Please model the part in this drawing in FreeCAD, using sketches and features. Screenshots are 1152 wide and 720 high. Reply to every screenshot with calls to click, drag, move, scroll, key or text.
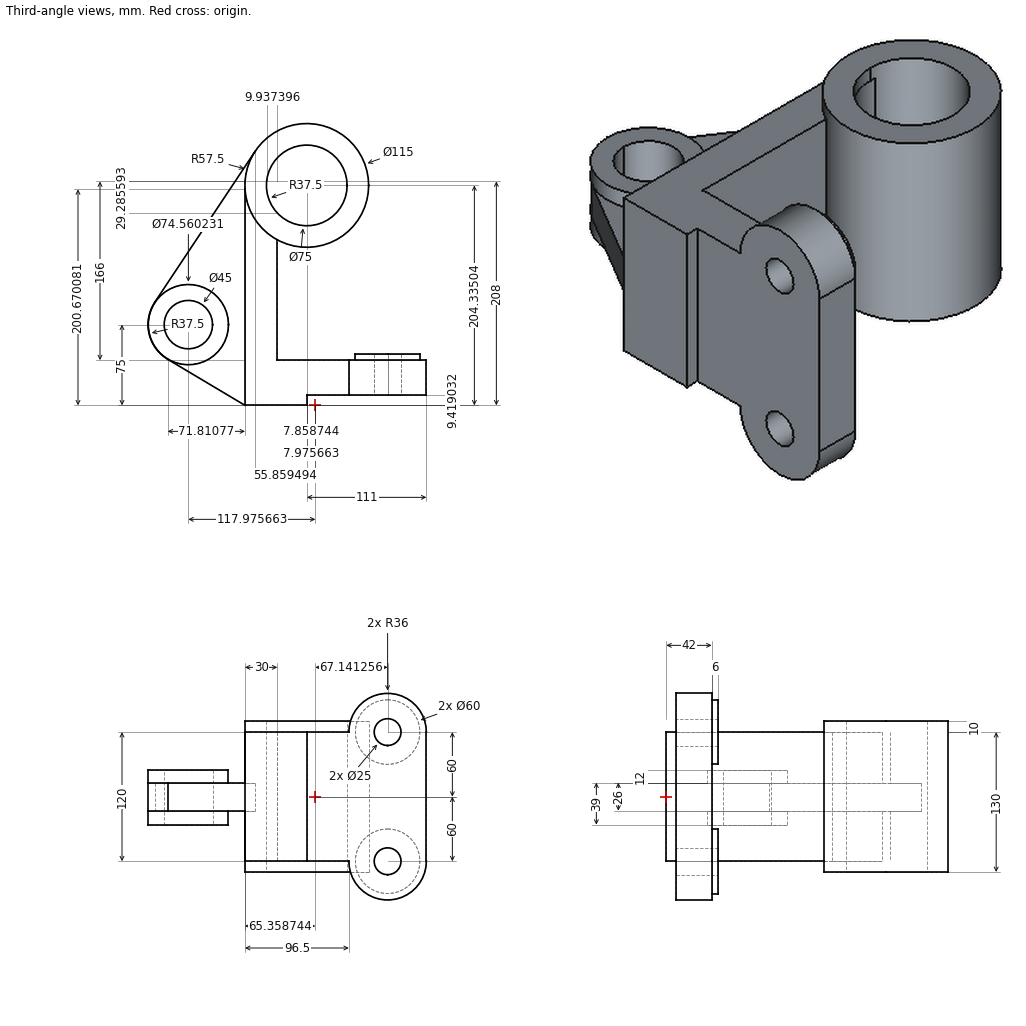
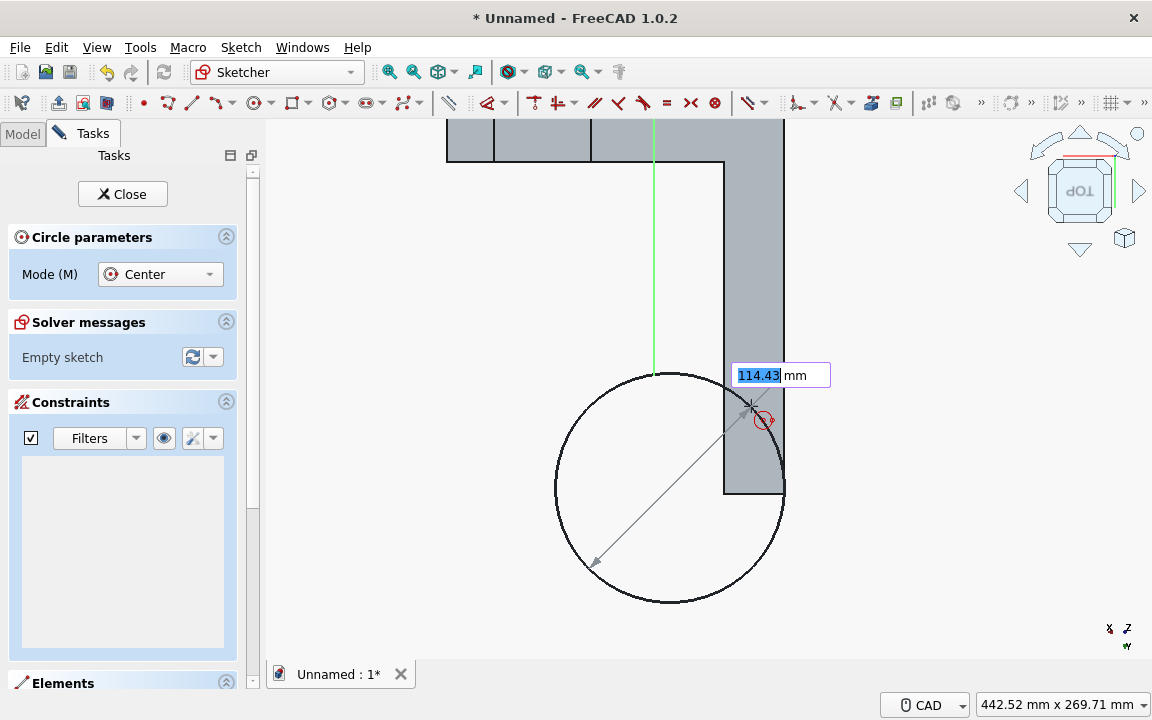
text(115)
key(Return)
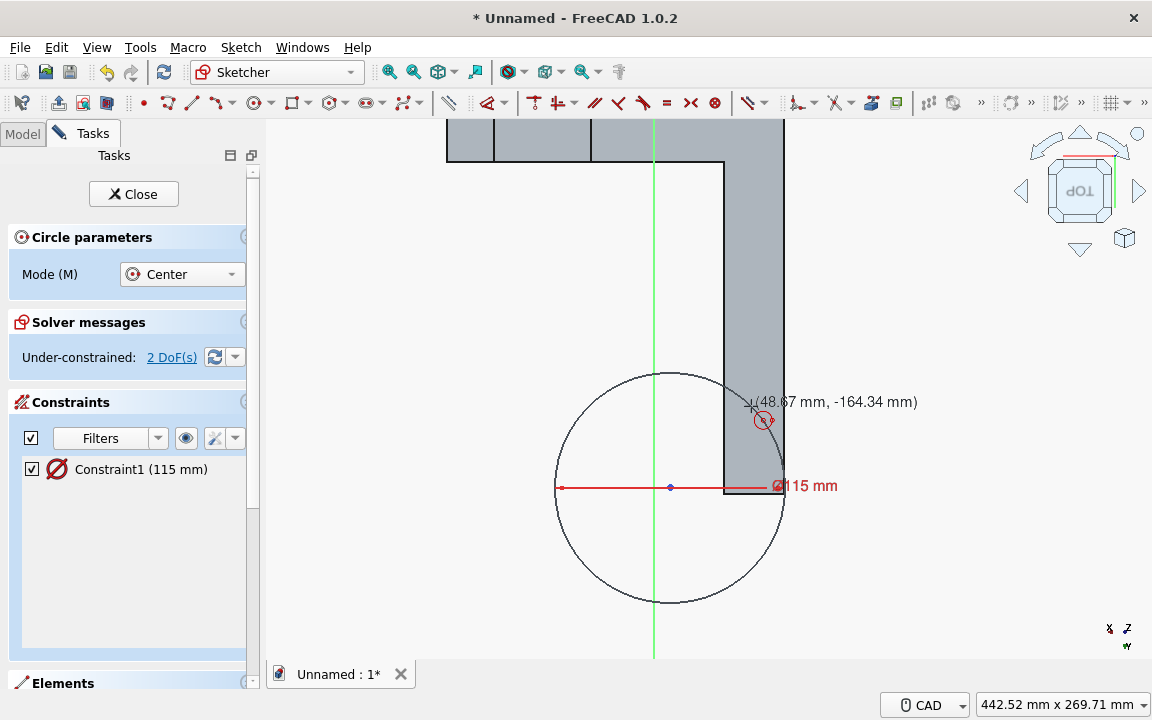
click(670, 488)
move(723, 434)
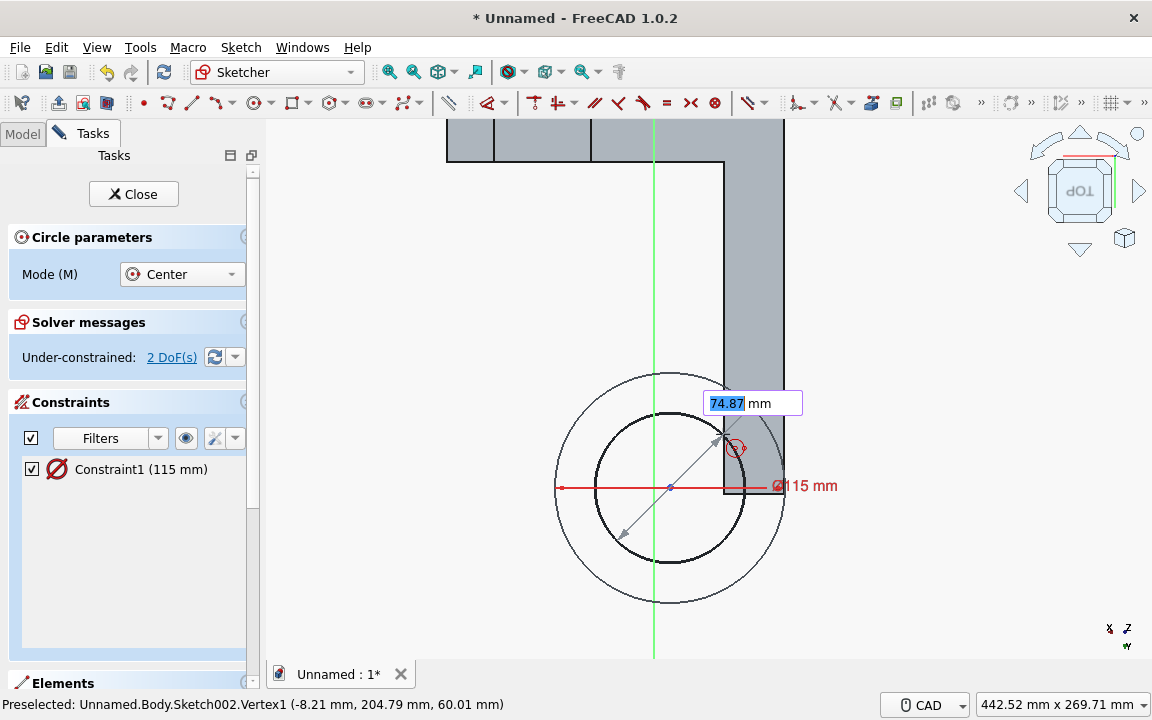
text(75)
key(Return)
key(Escape)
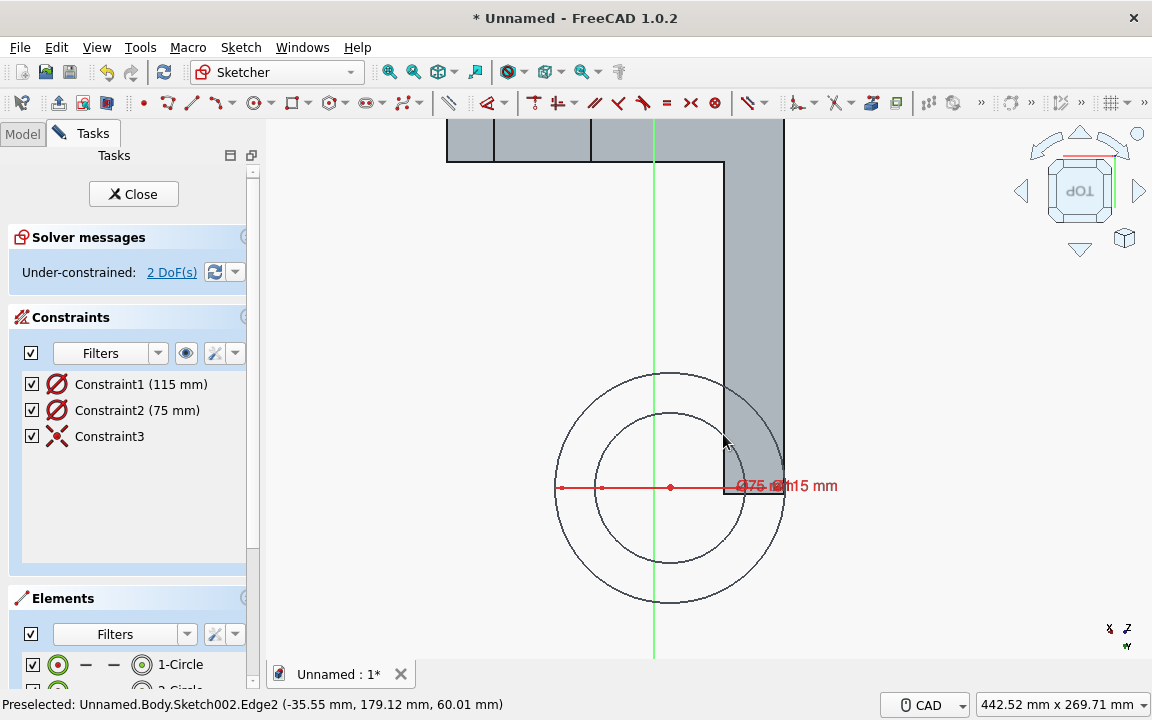
click(488, 104)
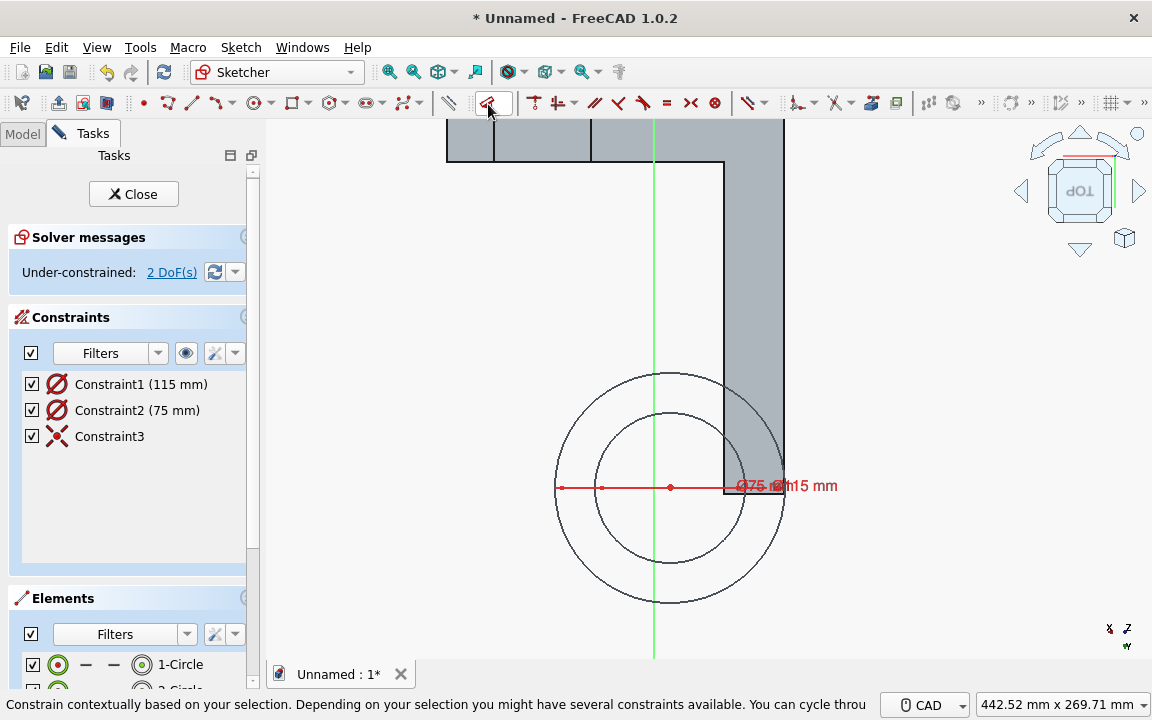
scroll(670, 488, up, 5)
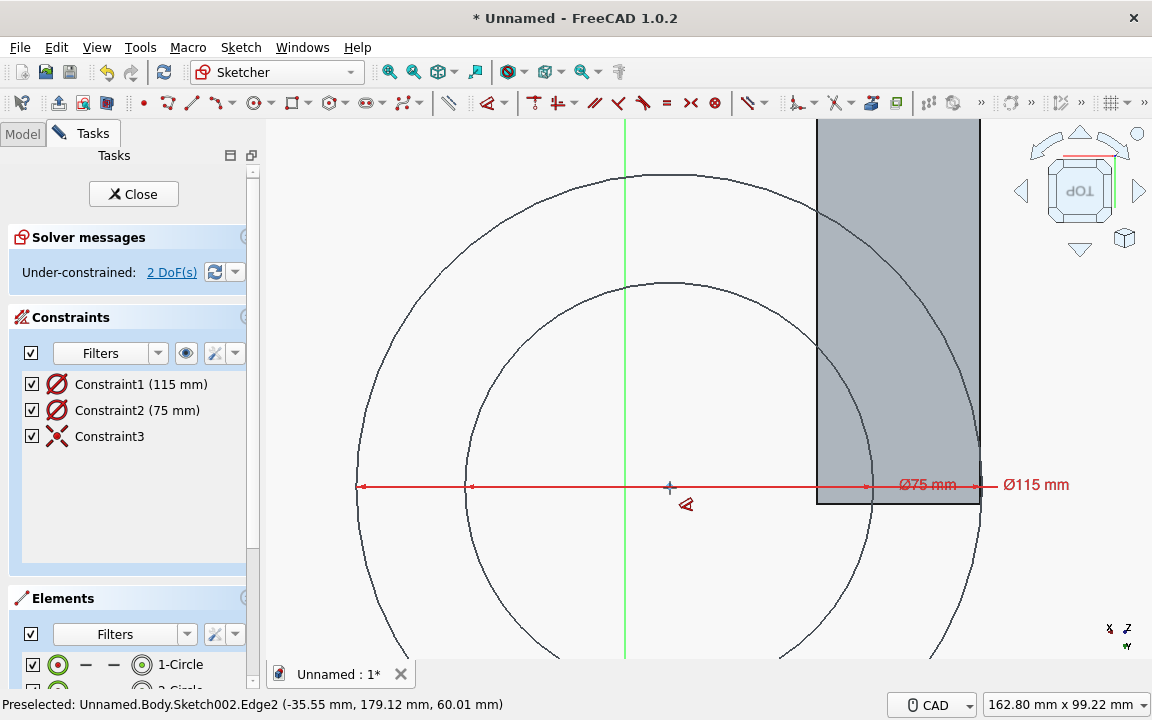
click(669, 487)
click(647, 521)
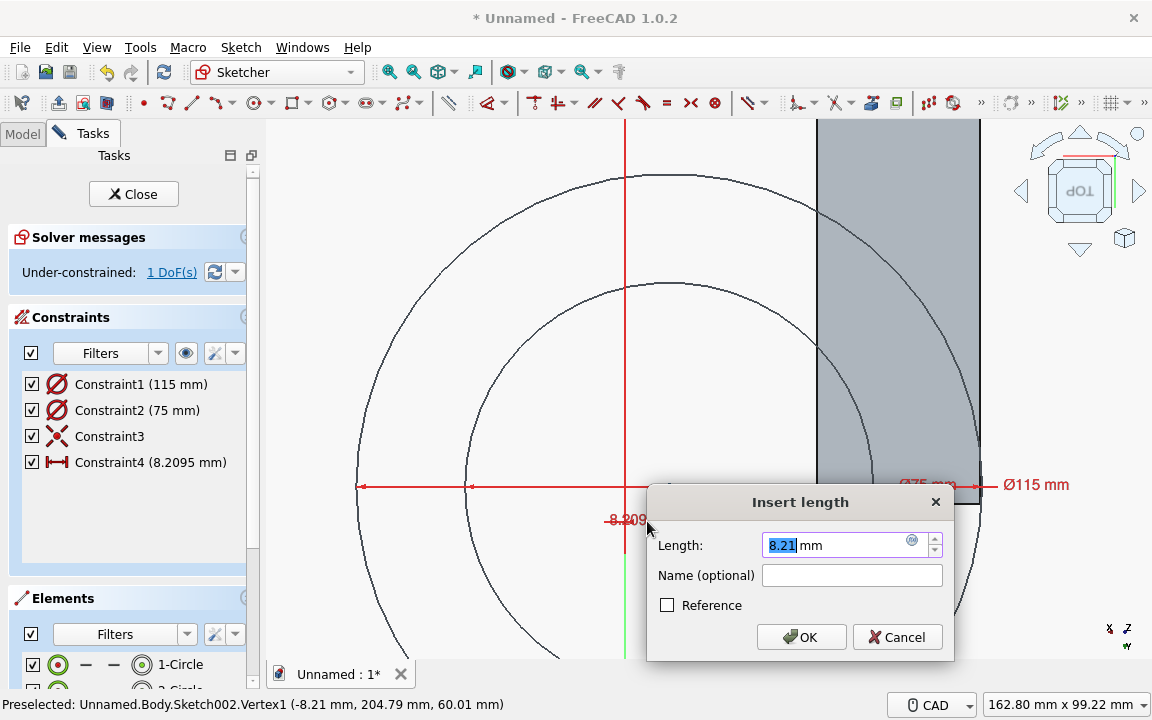
text(7.975663)
key(Return)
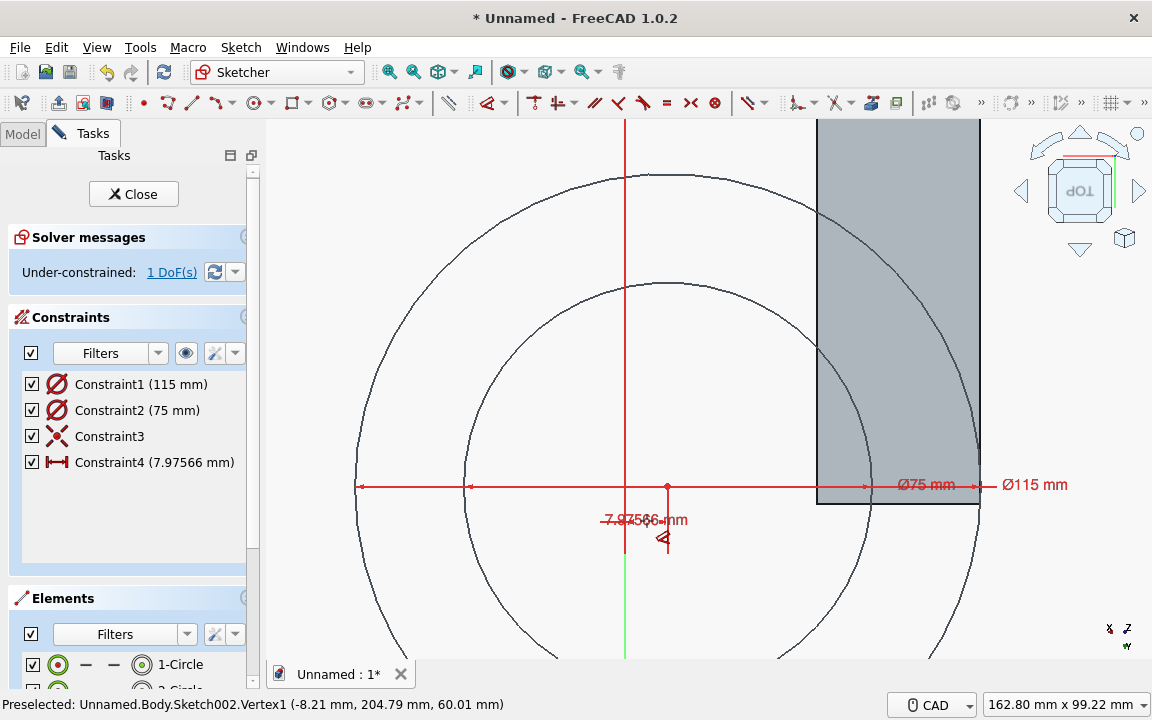
scroll(632, 489, down, 7)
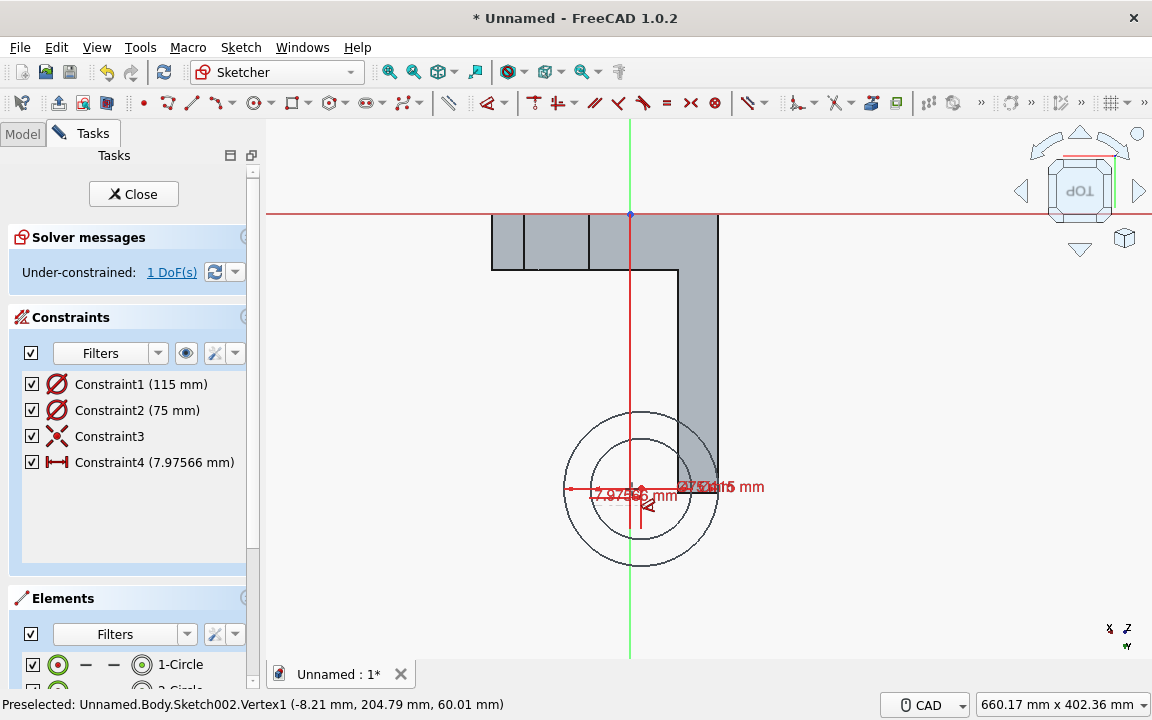
click(641, 489)
click(596, 352)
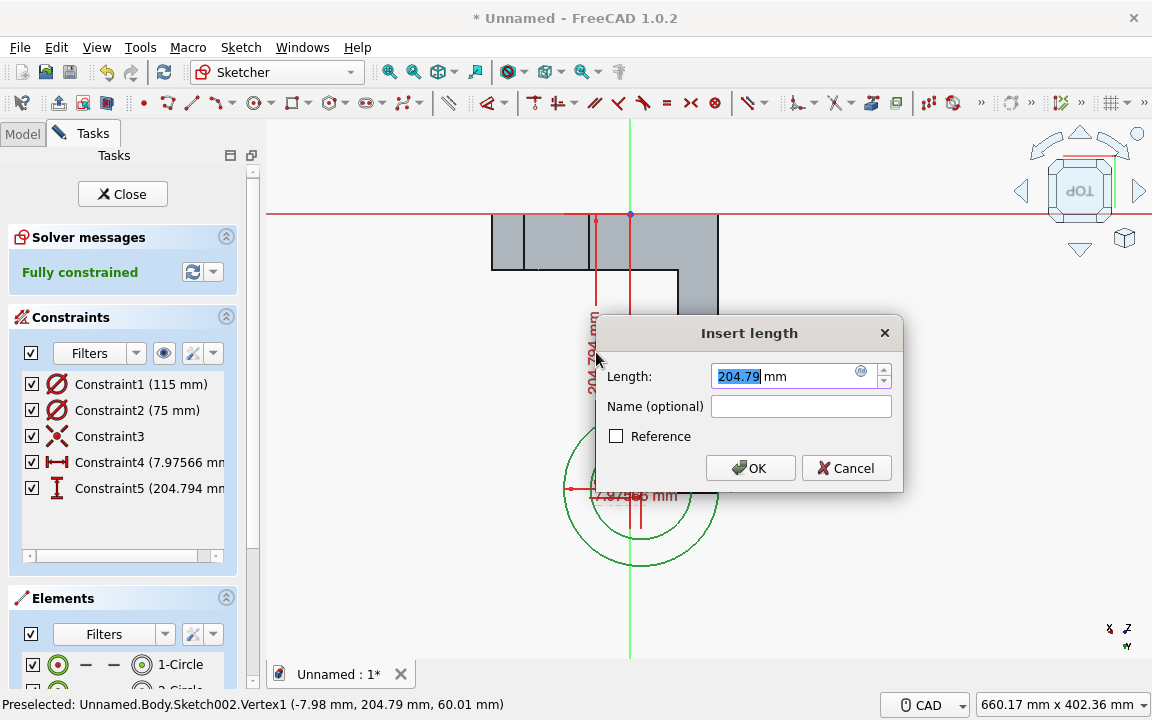
text(204.33504)
key(Return)
key(Escape)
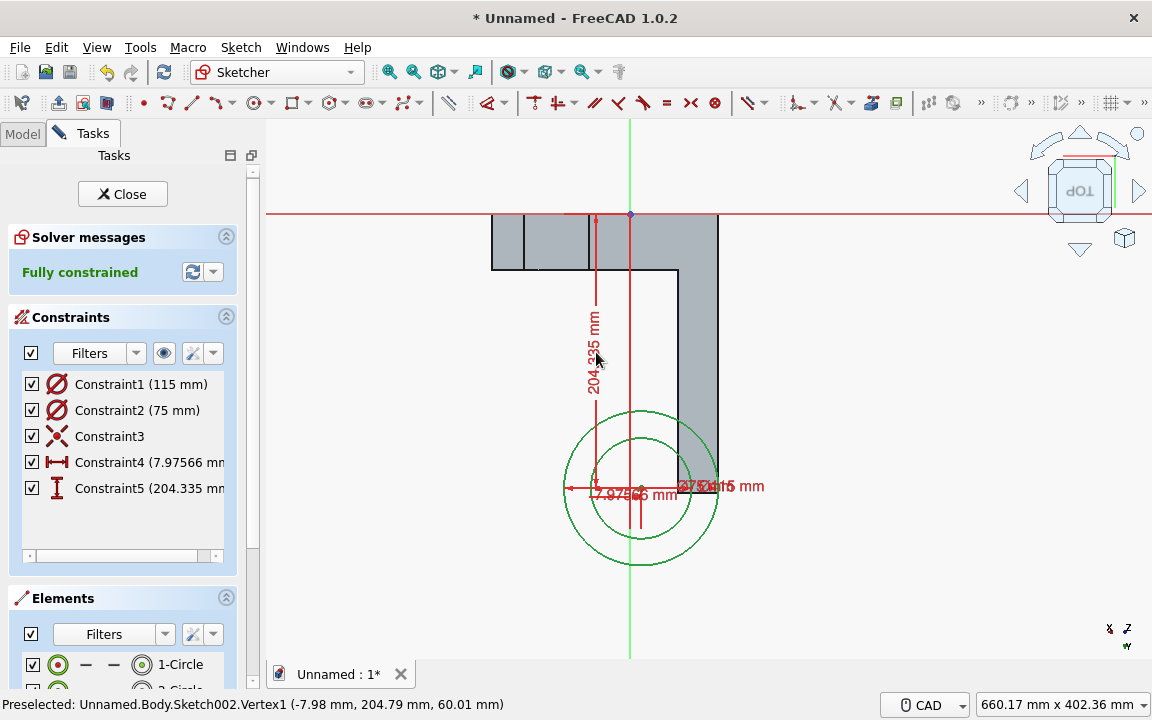
click(123, 194)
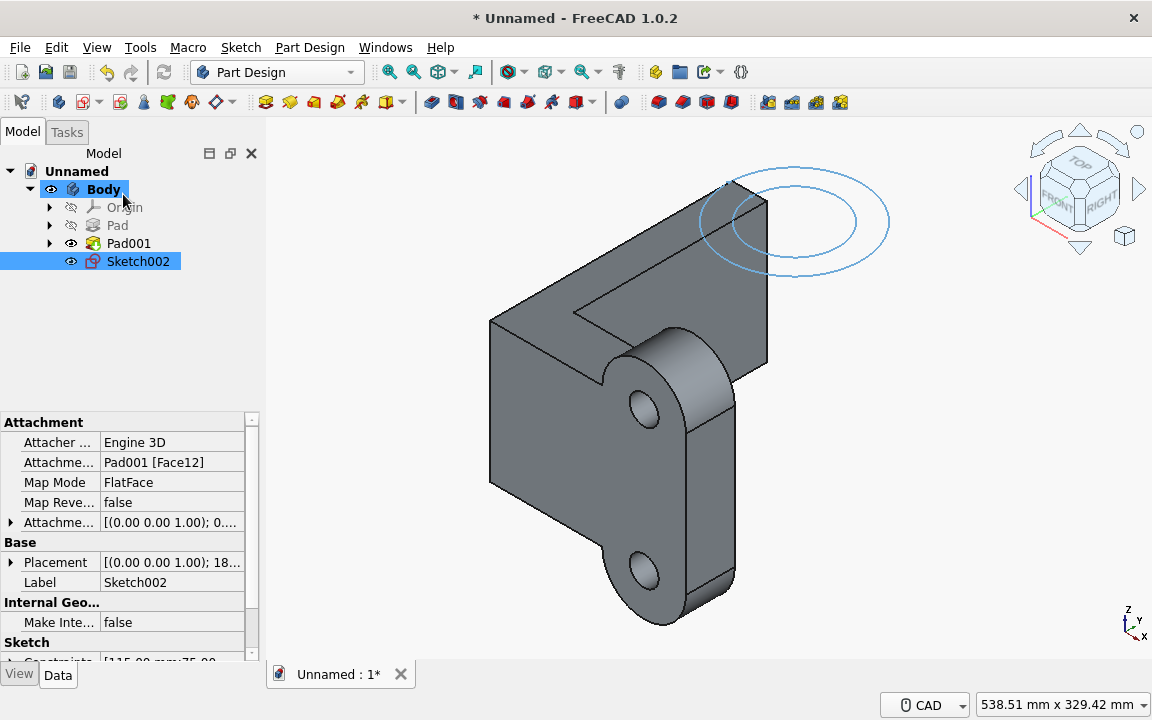
click(266, 102)